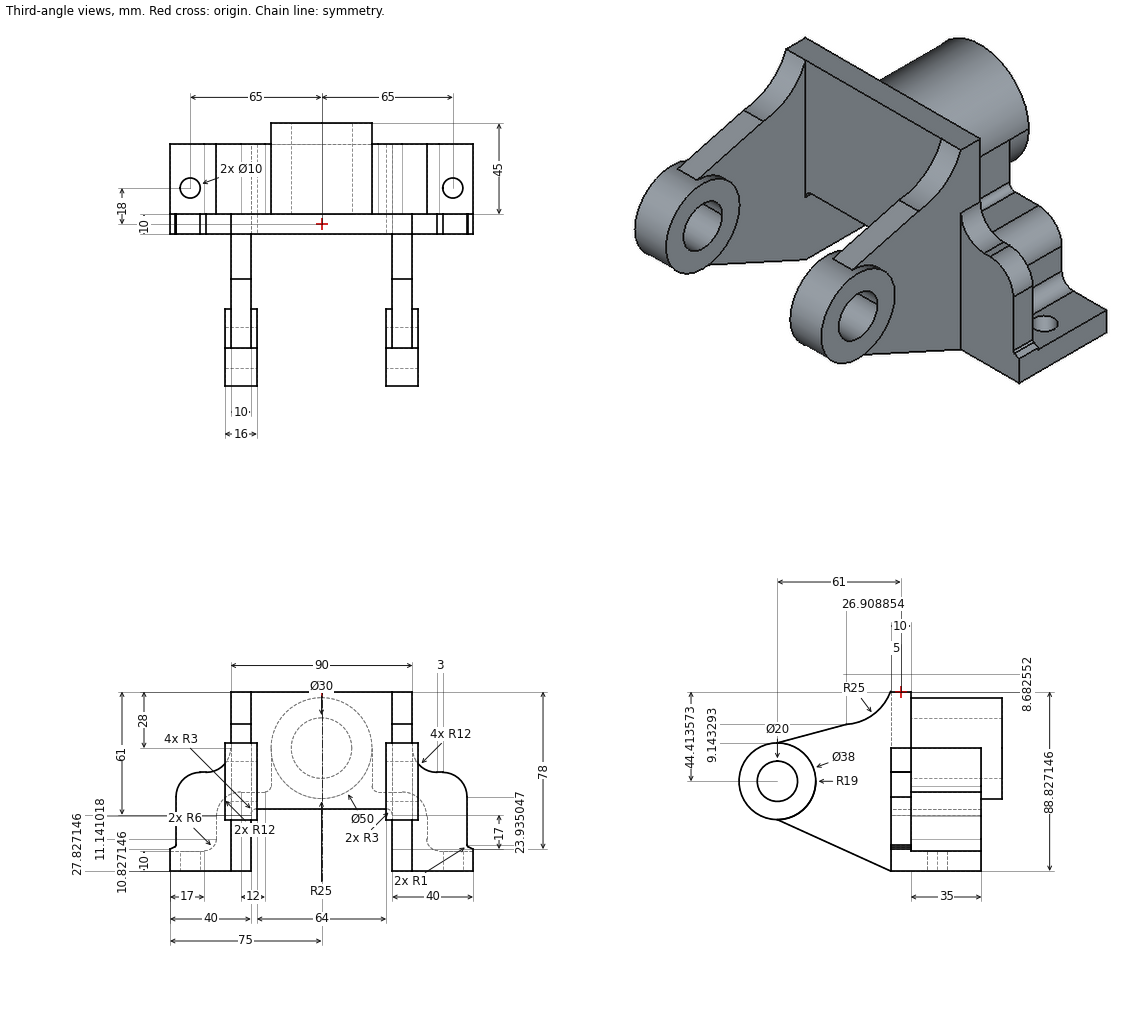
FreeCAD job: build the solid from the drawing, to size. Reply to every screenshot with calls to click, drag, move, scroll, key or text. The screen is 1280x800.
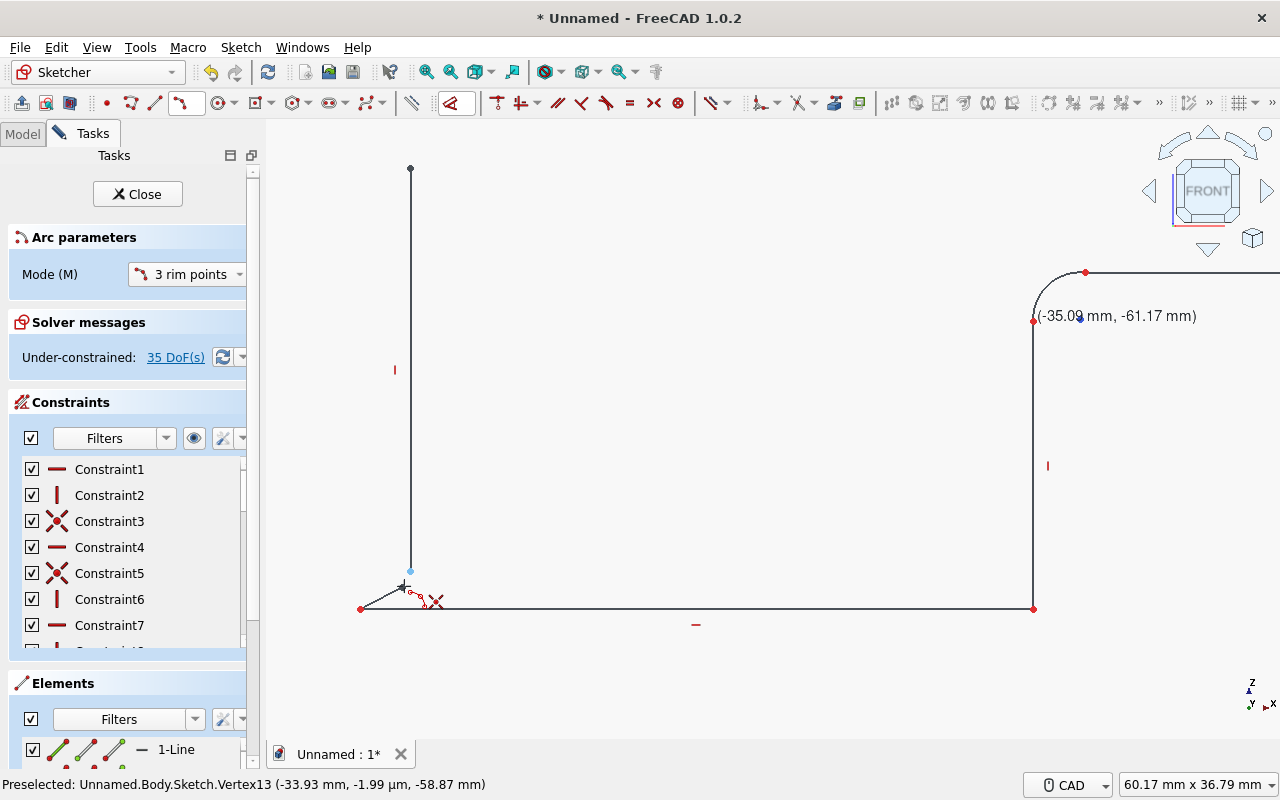
click(402, 587)
click(411, 571)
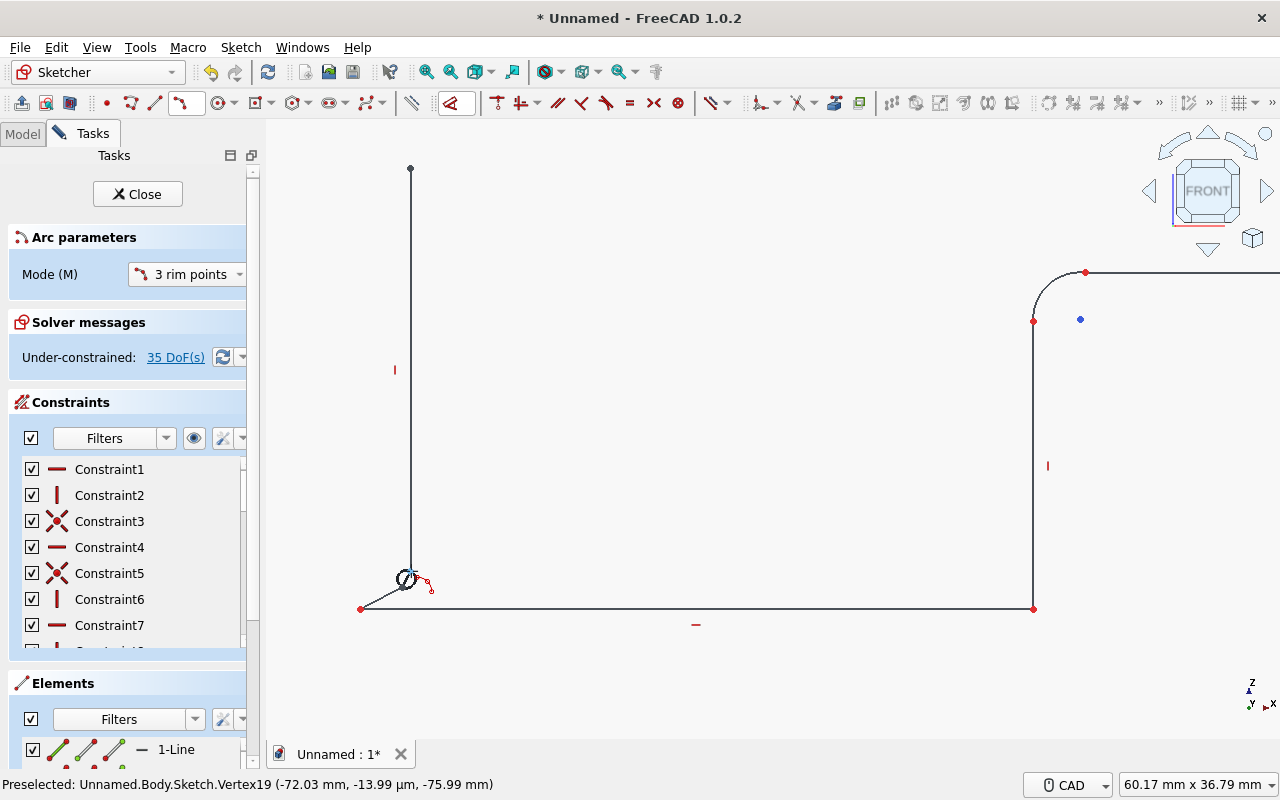
scroll(409, 579, up, 10)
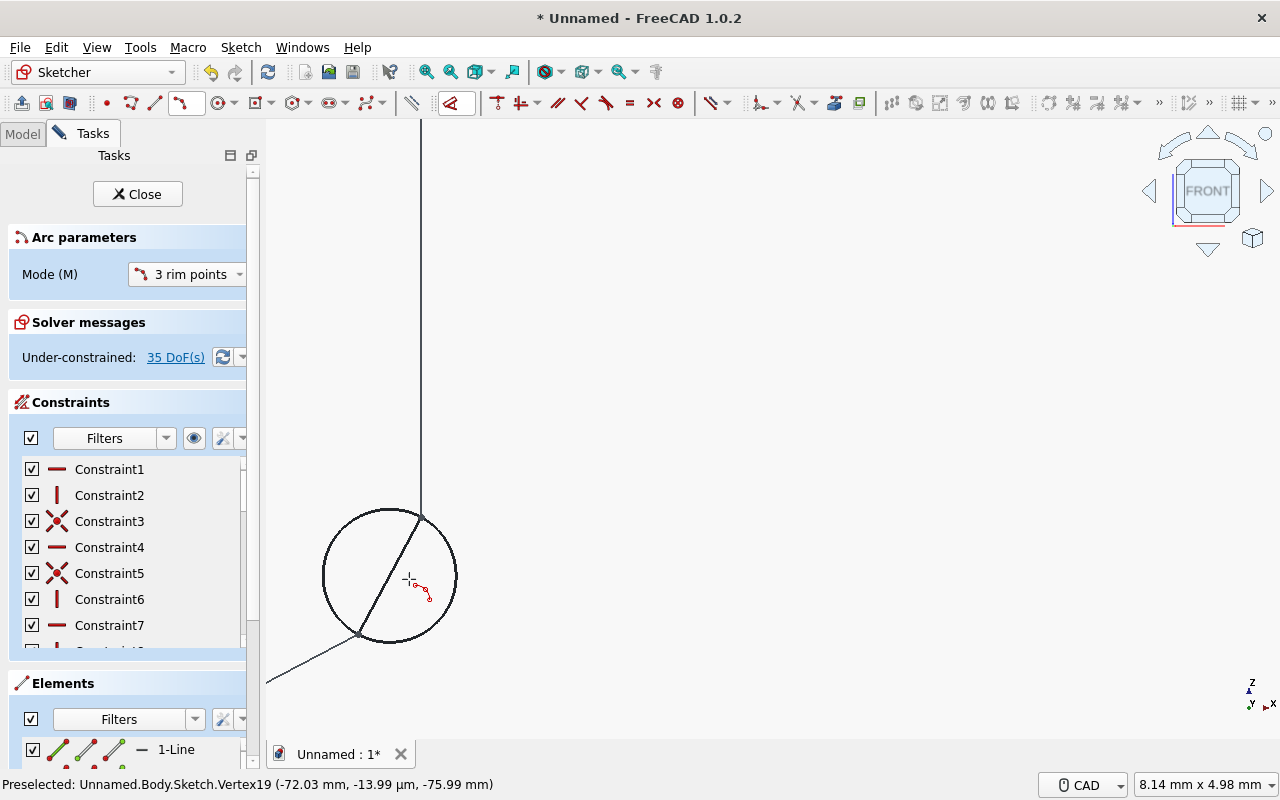
click(406, 576)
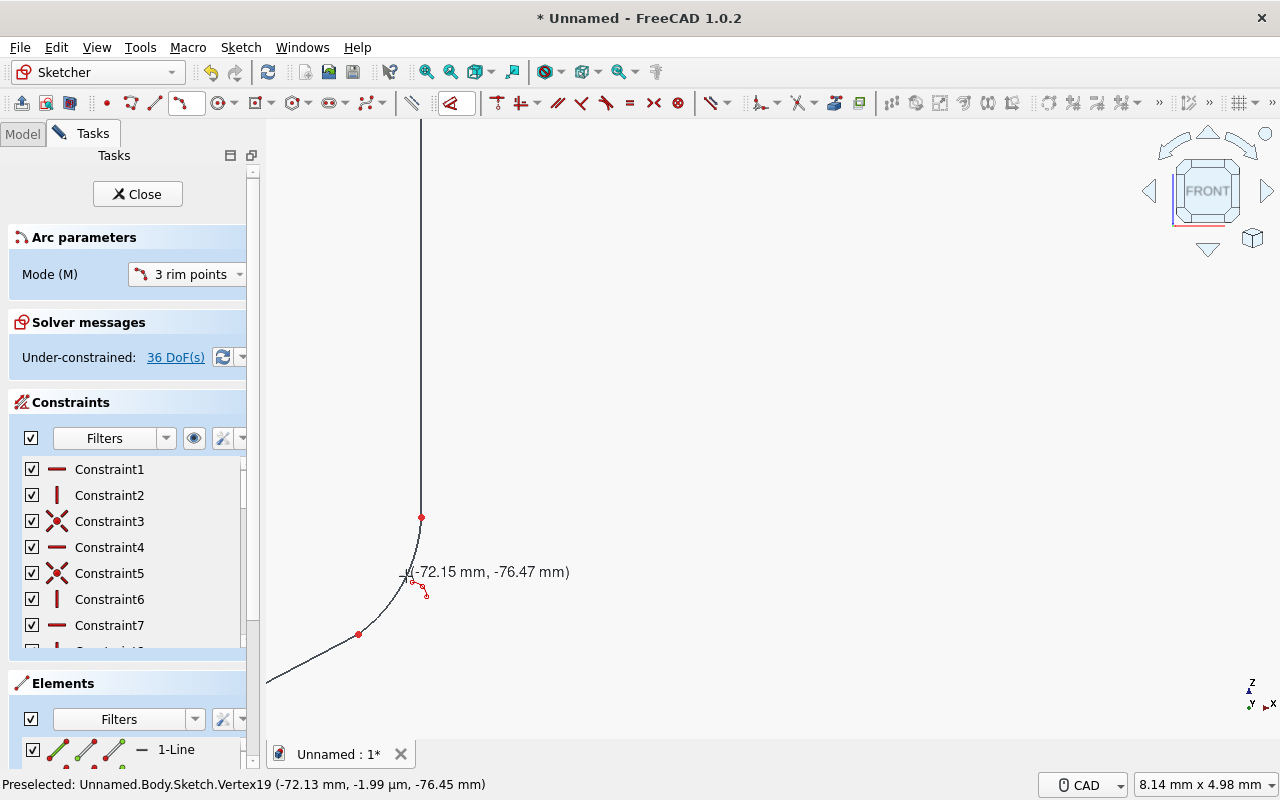
scroll(335, 621, down, 16)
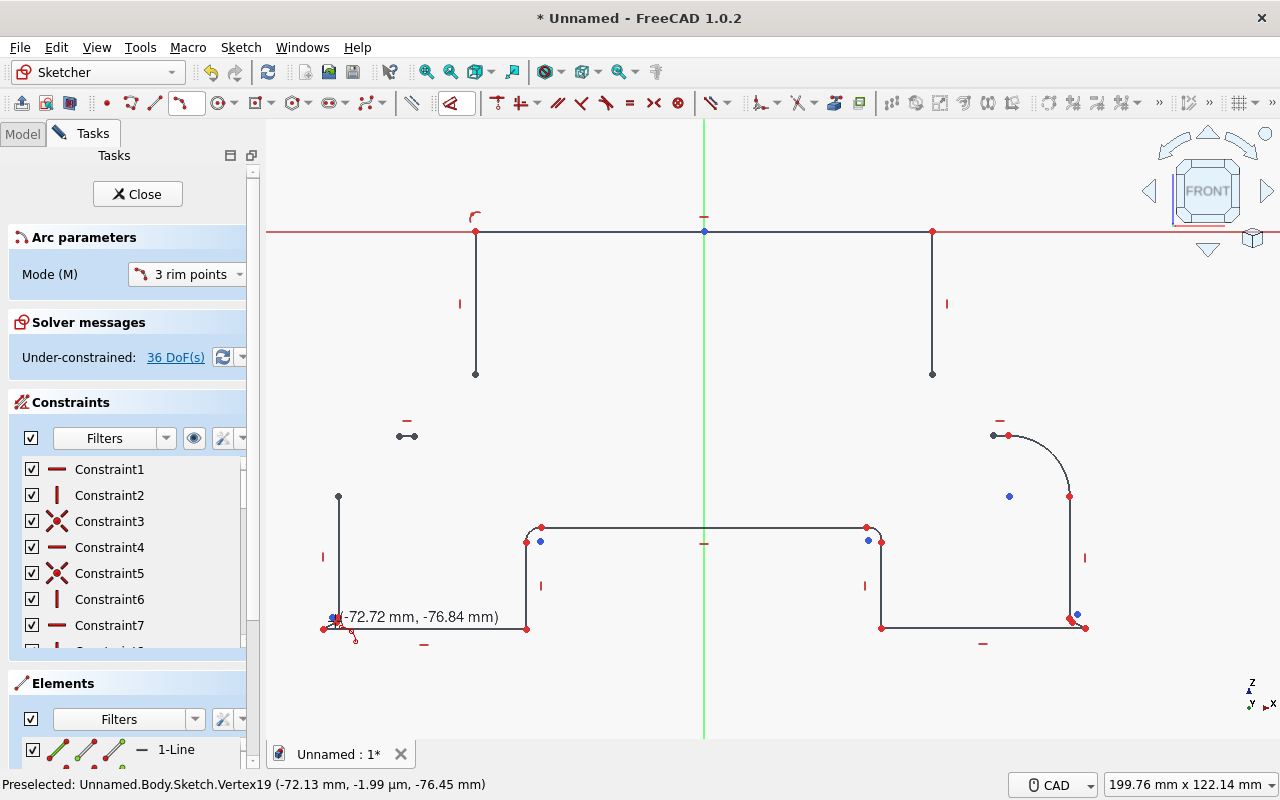
click(339, 496)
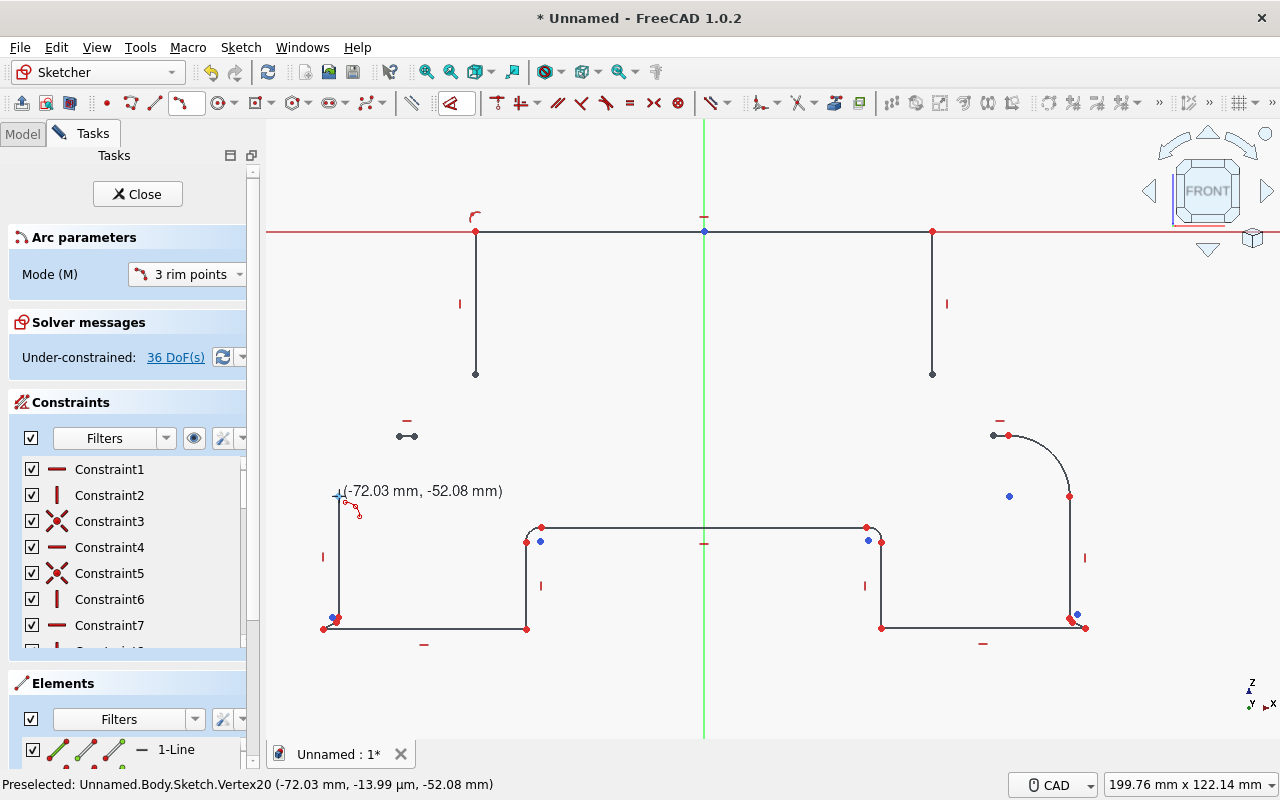
scroll(400, 435, up, 4)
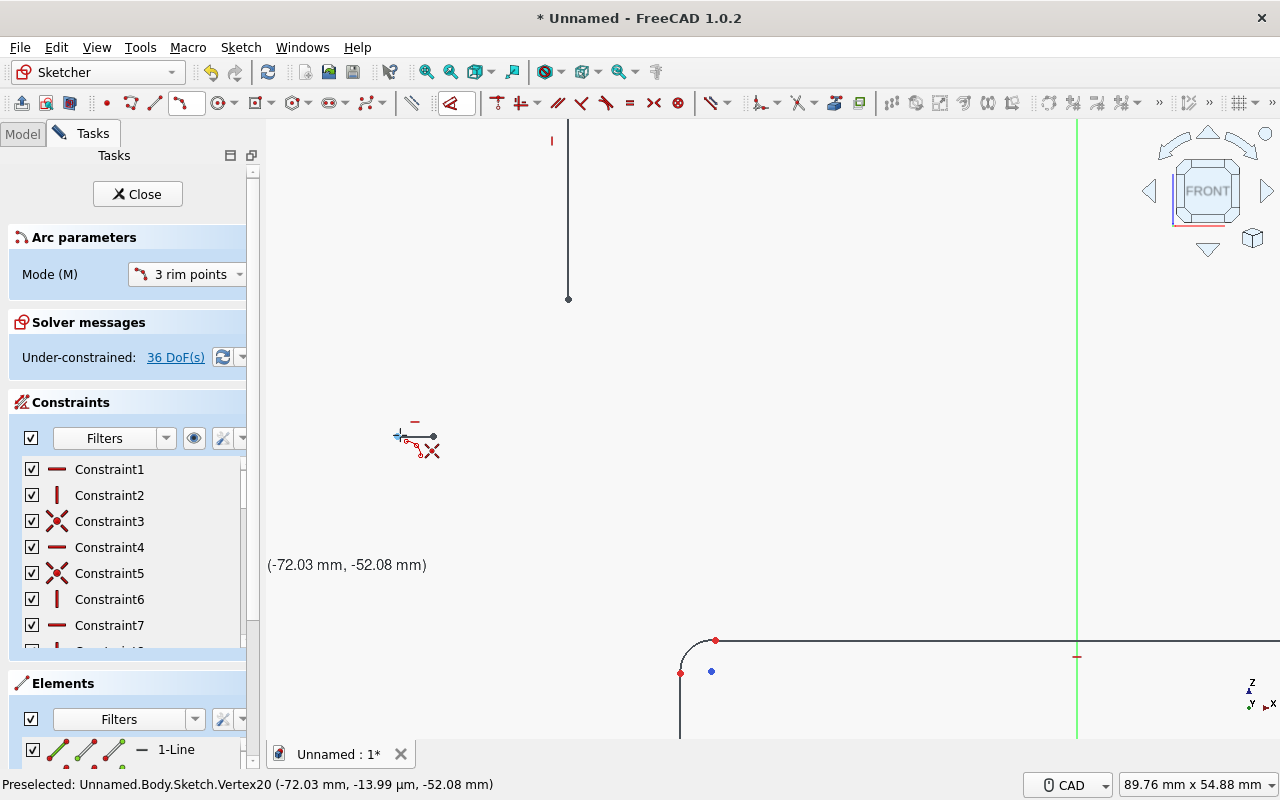
click(398, 437)
click(303, 474)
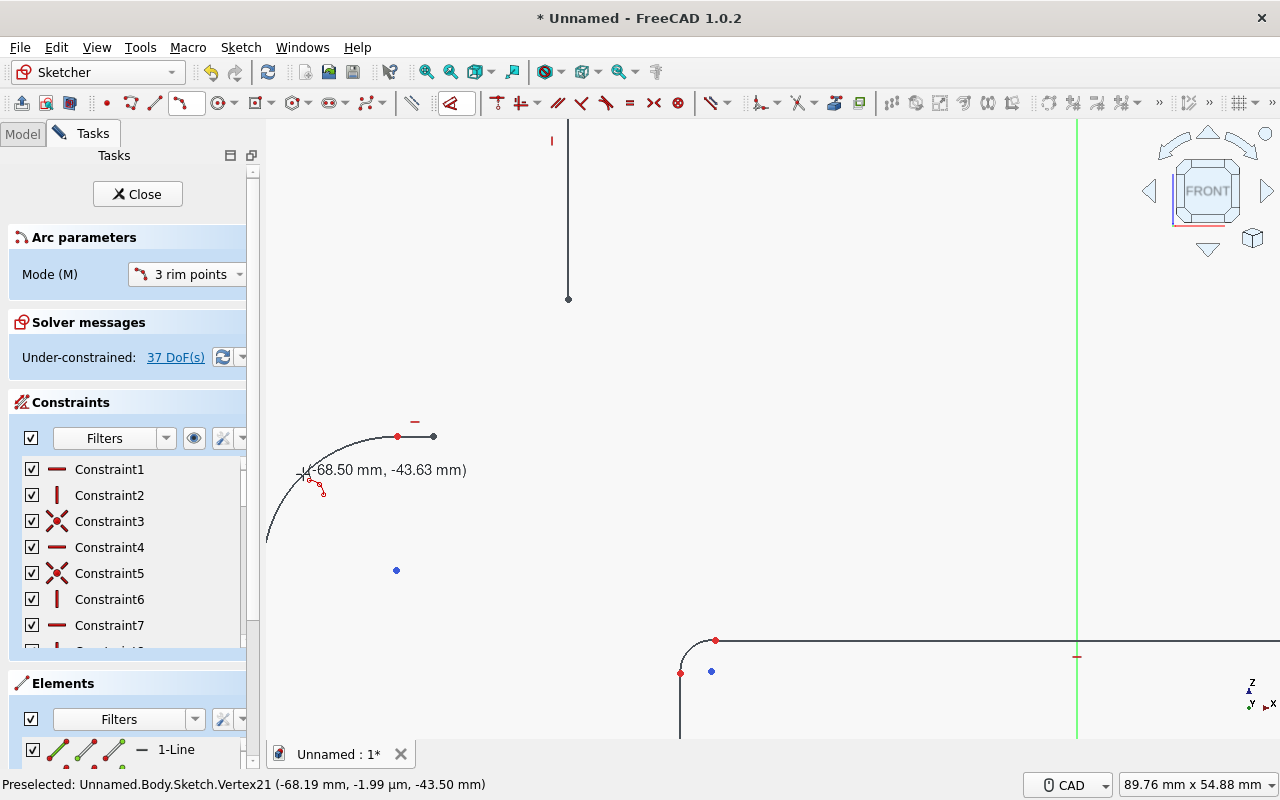
click(433, 437)
click(568, 300)
click(529, 394)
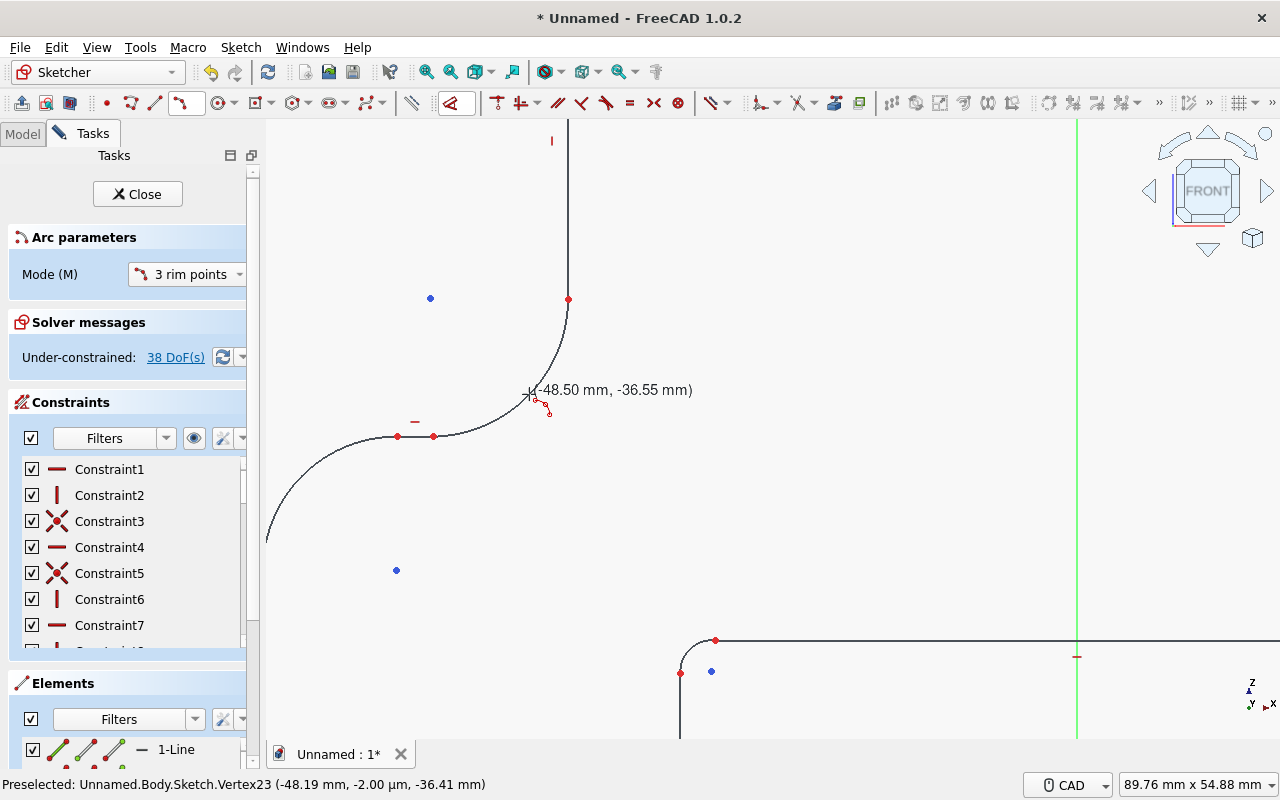
scroll(488, 433, down, 5)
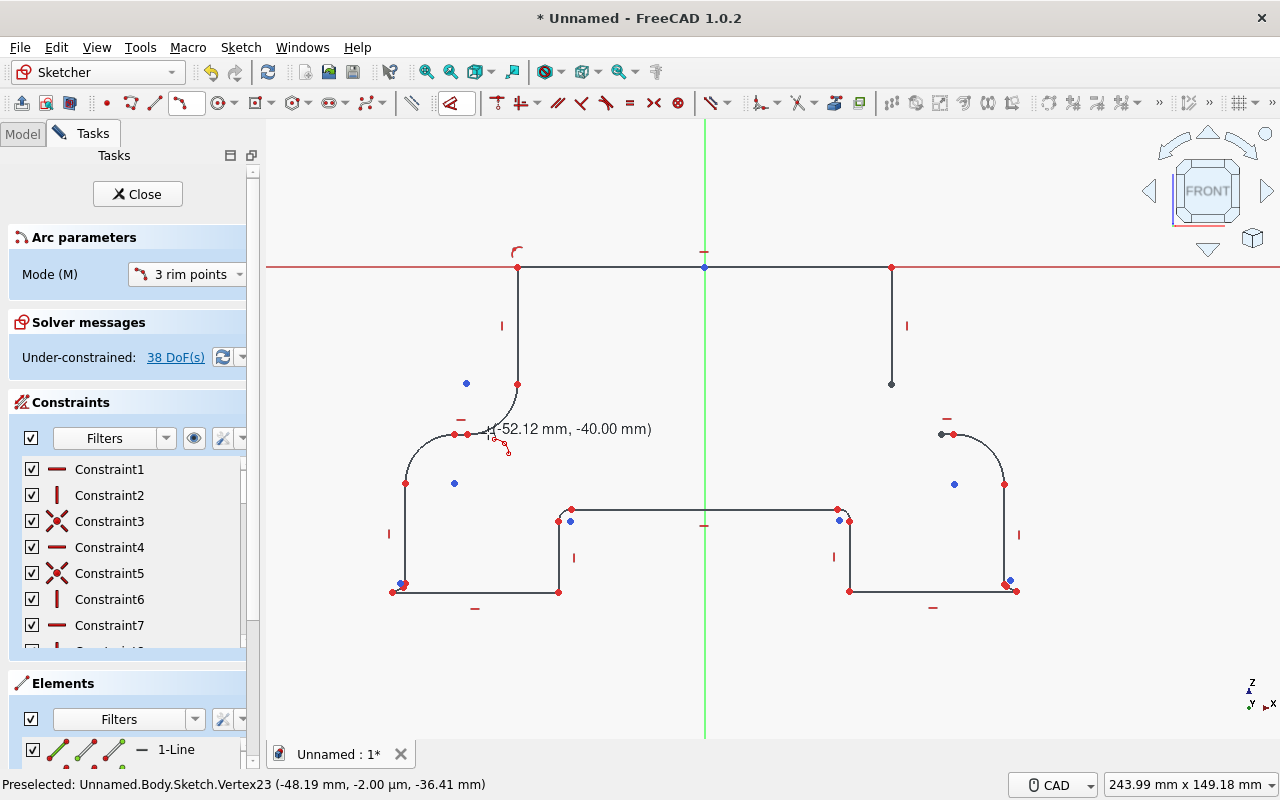
click(892, 384)